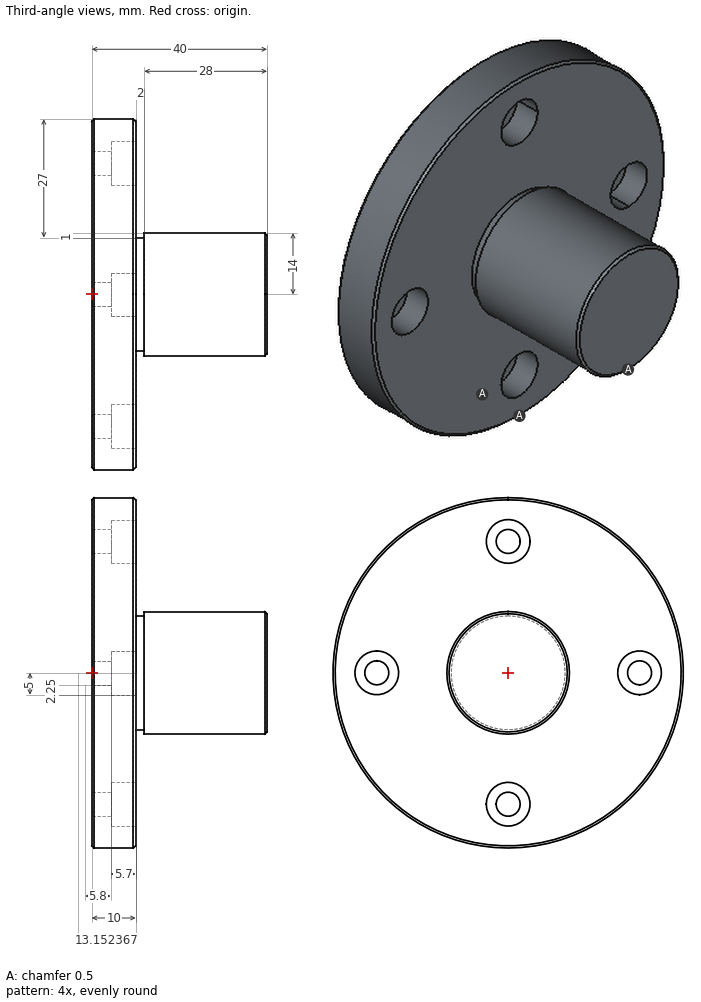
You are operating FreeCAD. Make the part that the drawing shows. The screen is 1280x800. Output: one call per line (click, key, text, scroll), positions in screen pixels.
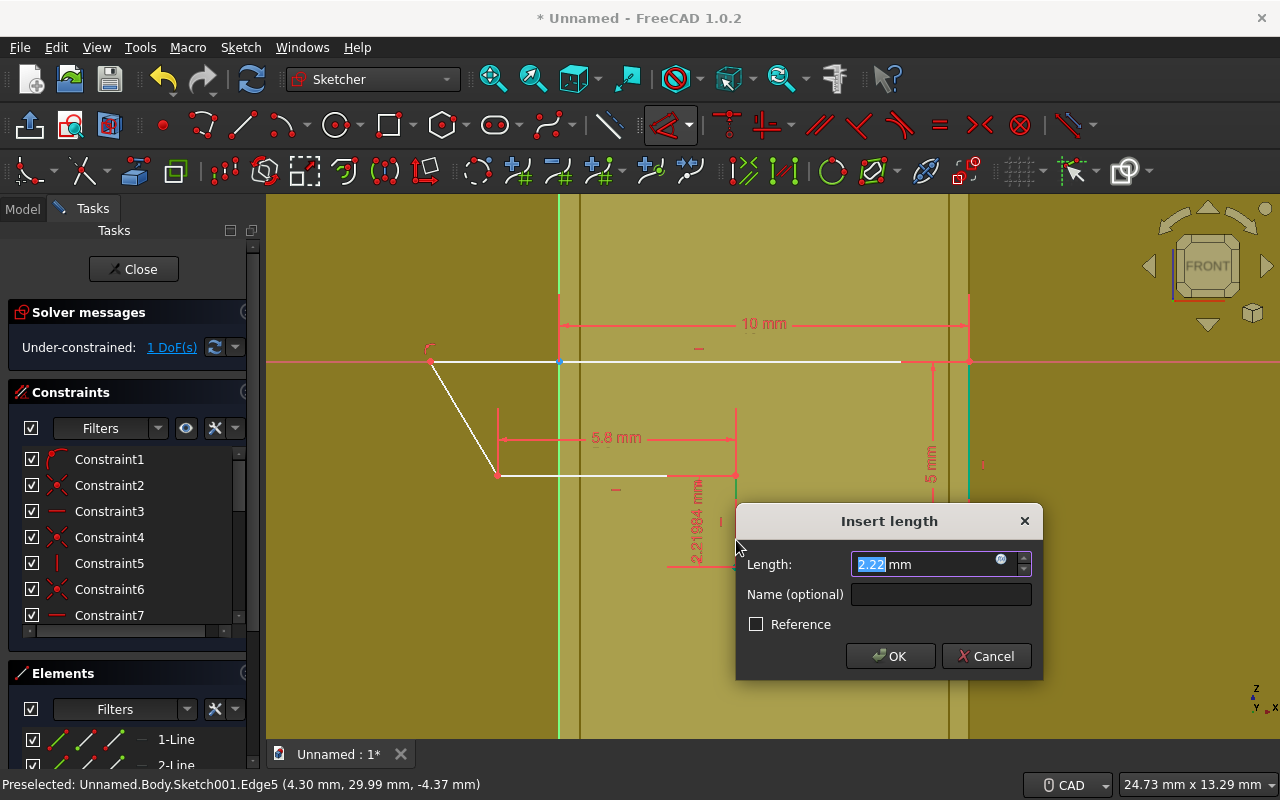
text(2.25)
key(Return)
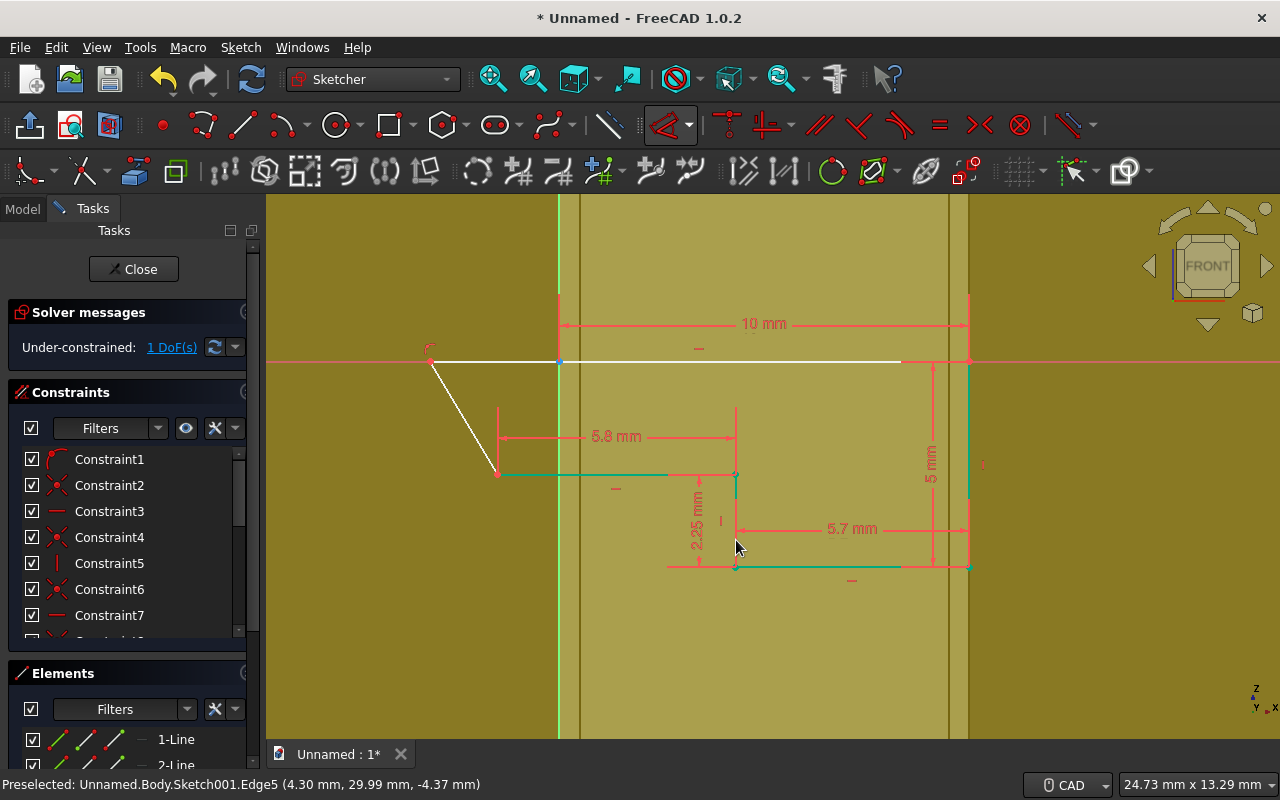
click(592, 362)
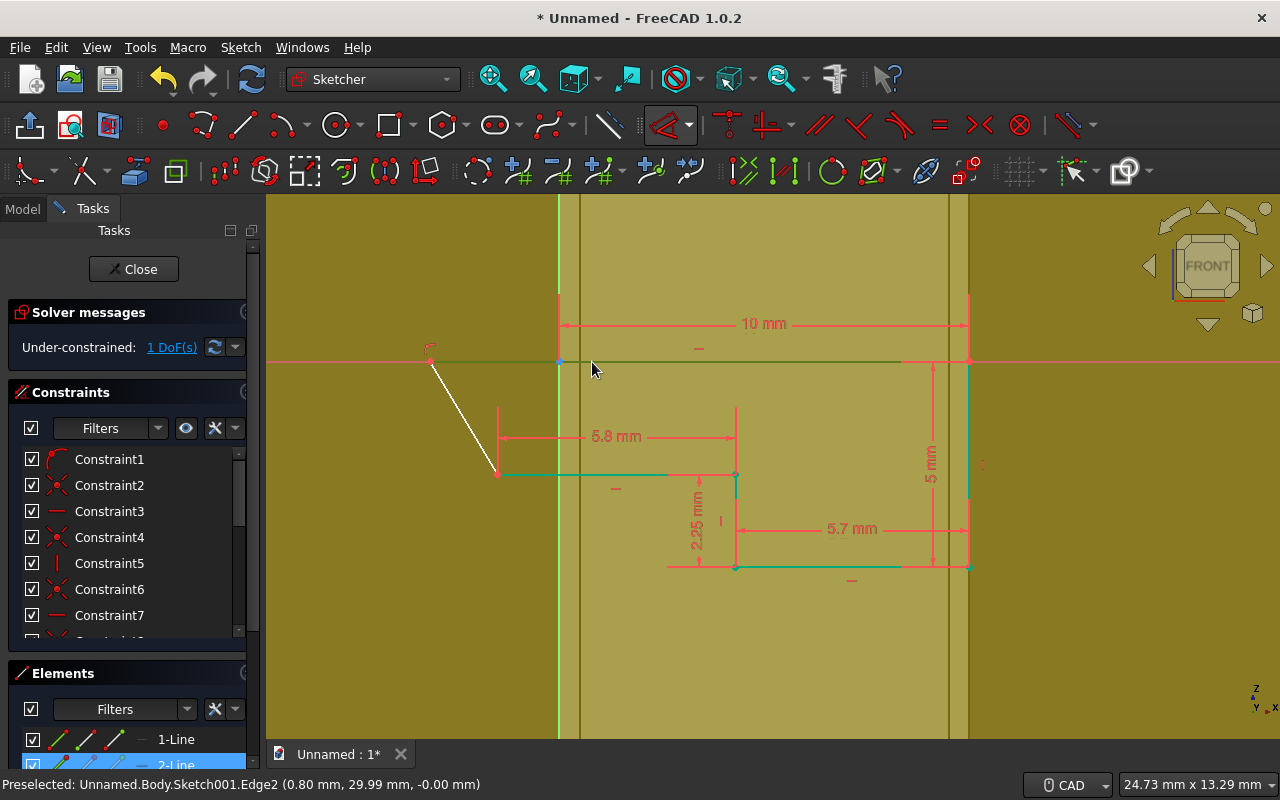
click(692, 126)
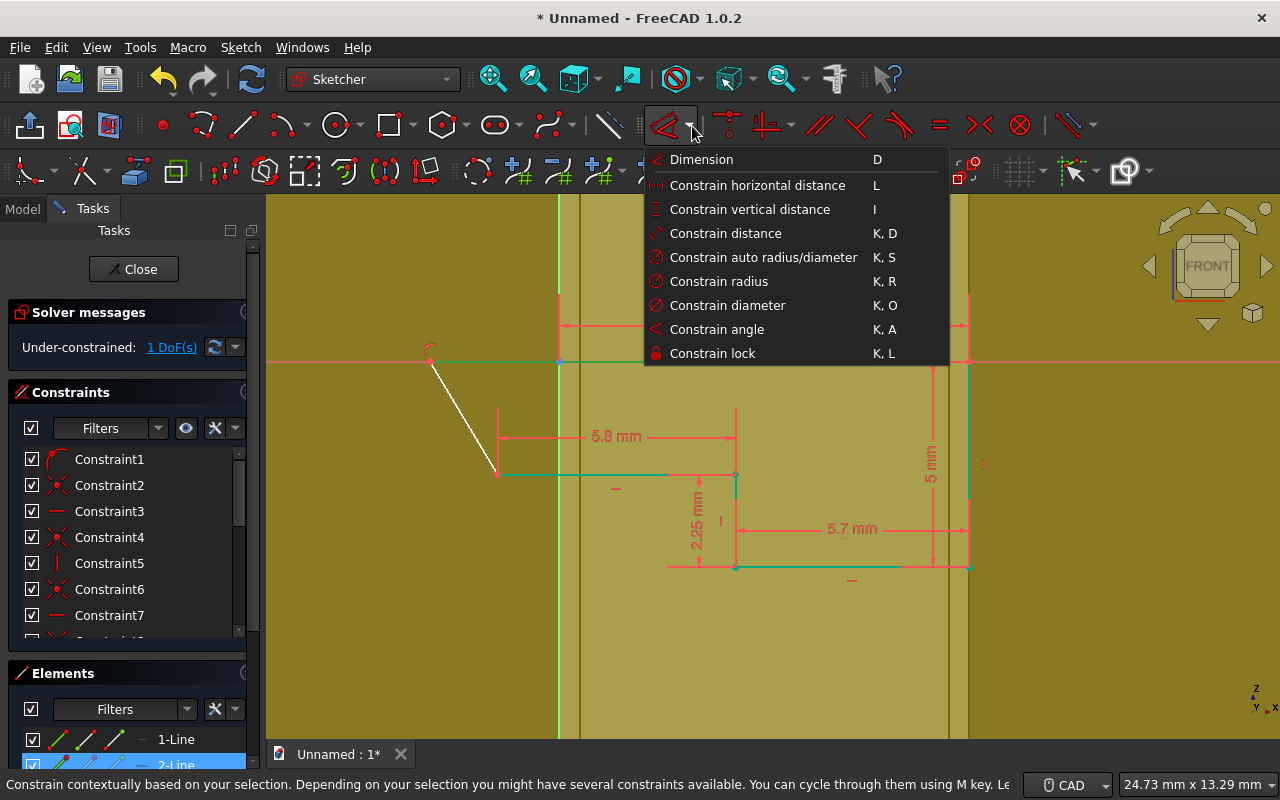
click(797, 185)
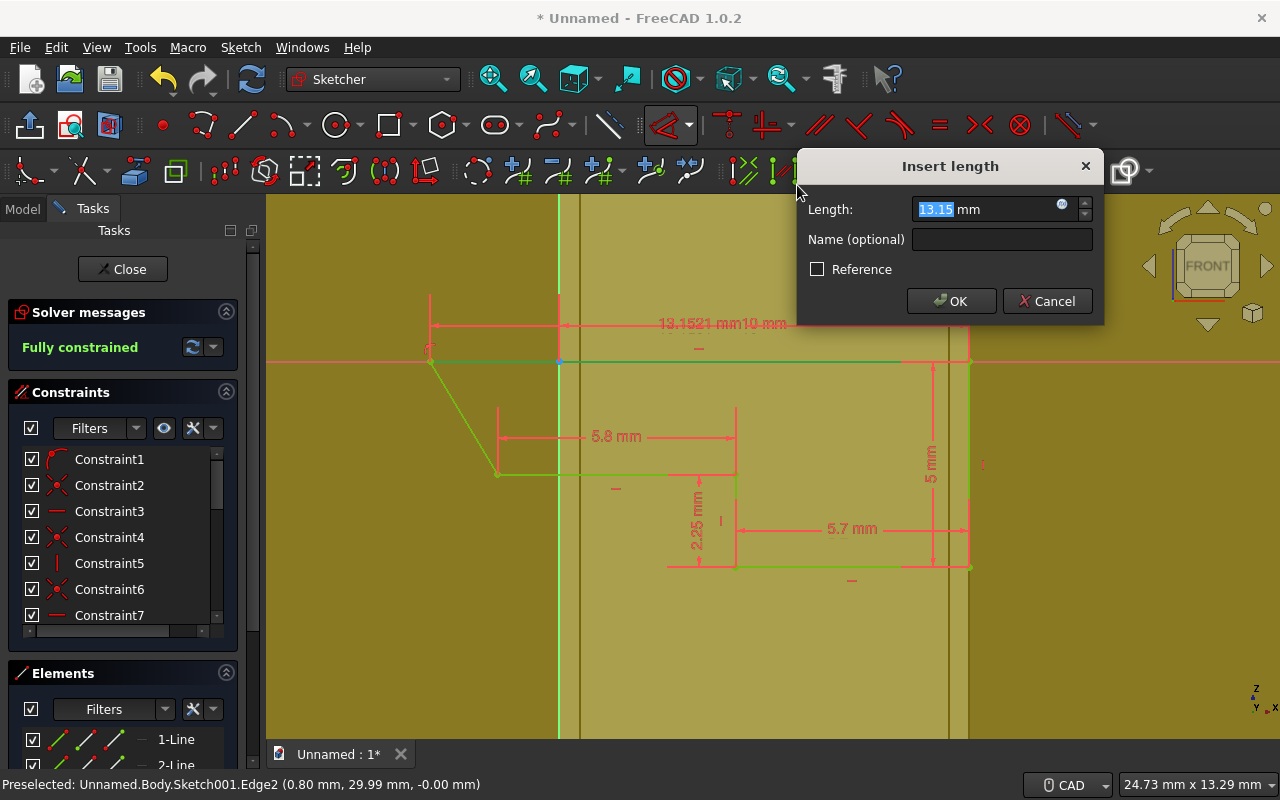
text(13.152367)
key(Return)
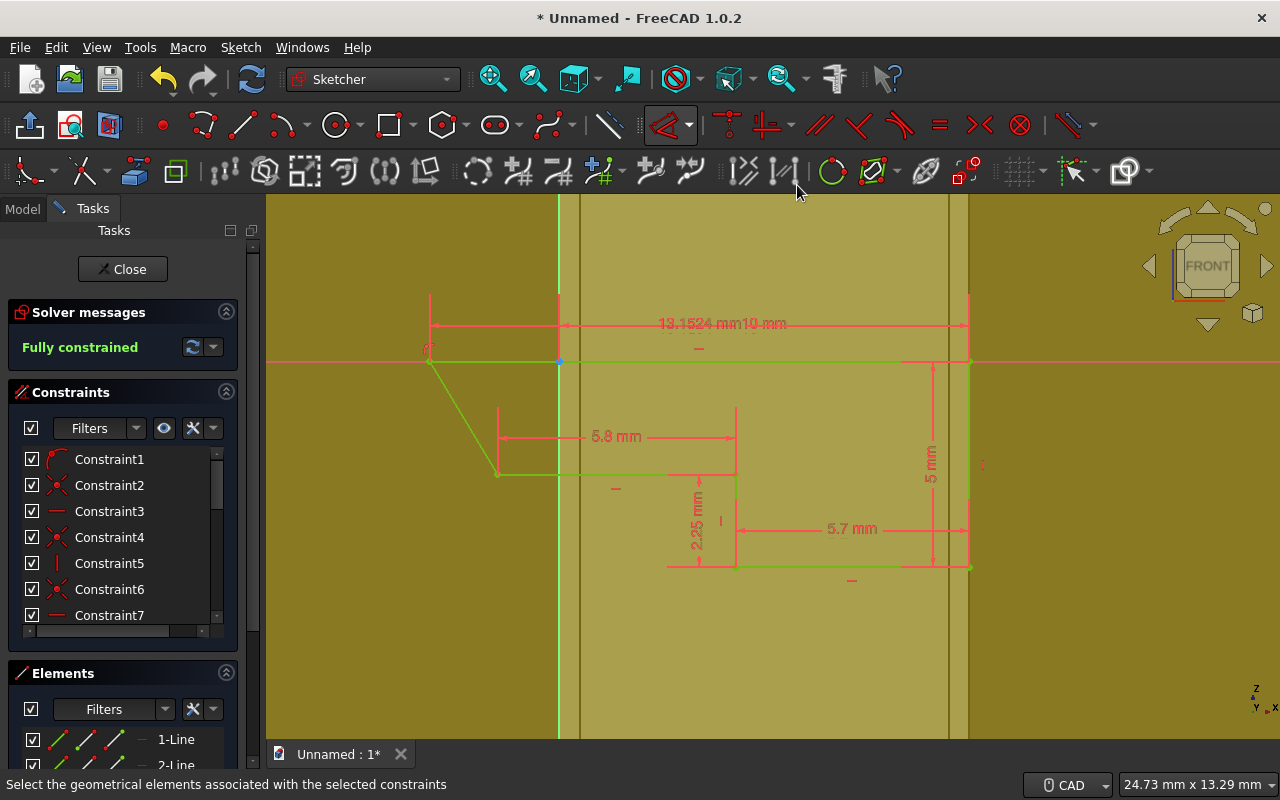
click(123, 269)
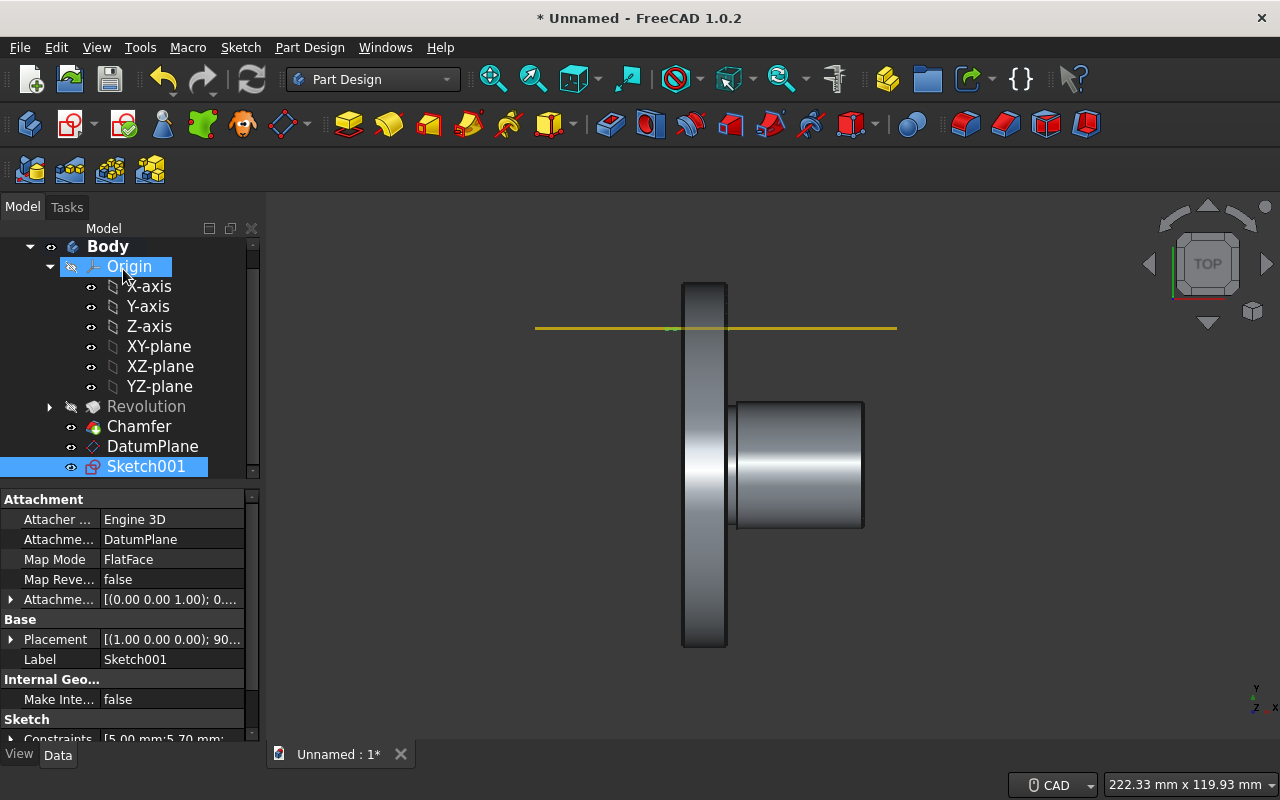
click(692, 124)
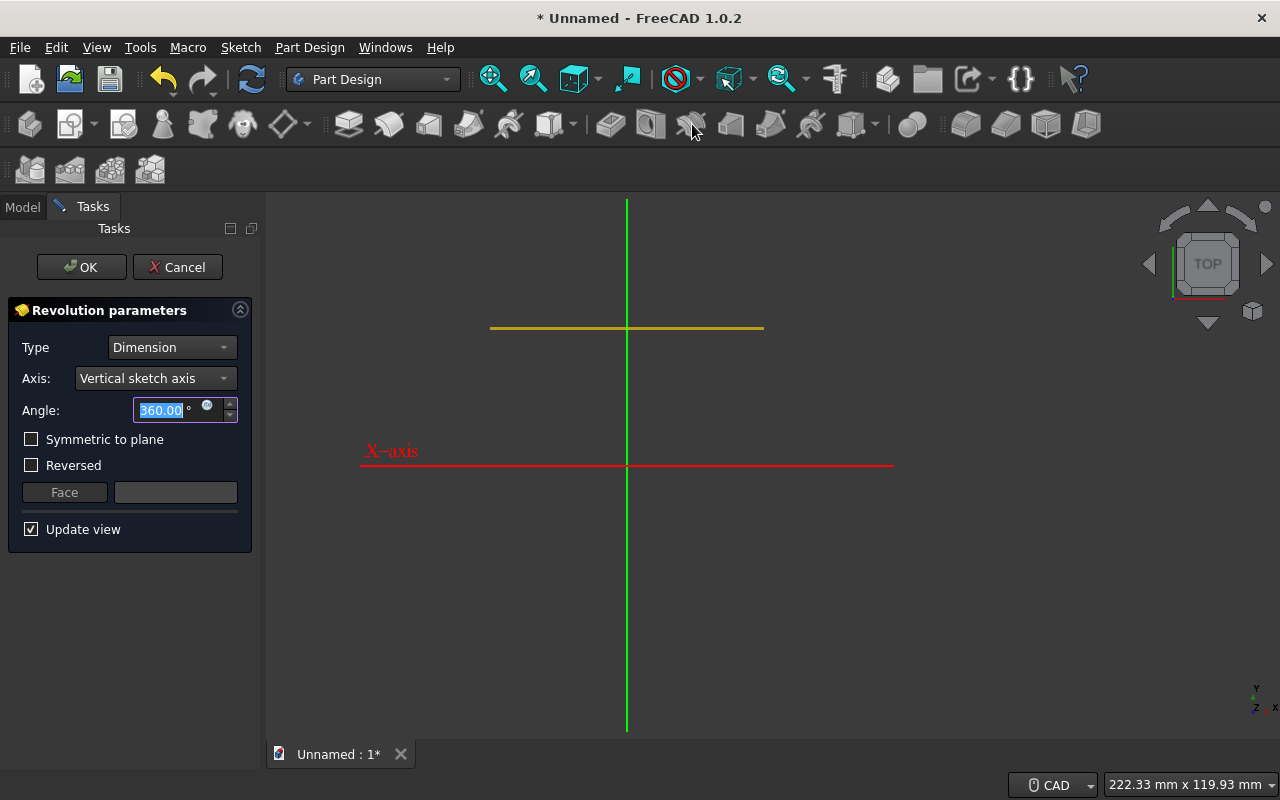
click(156, 378)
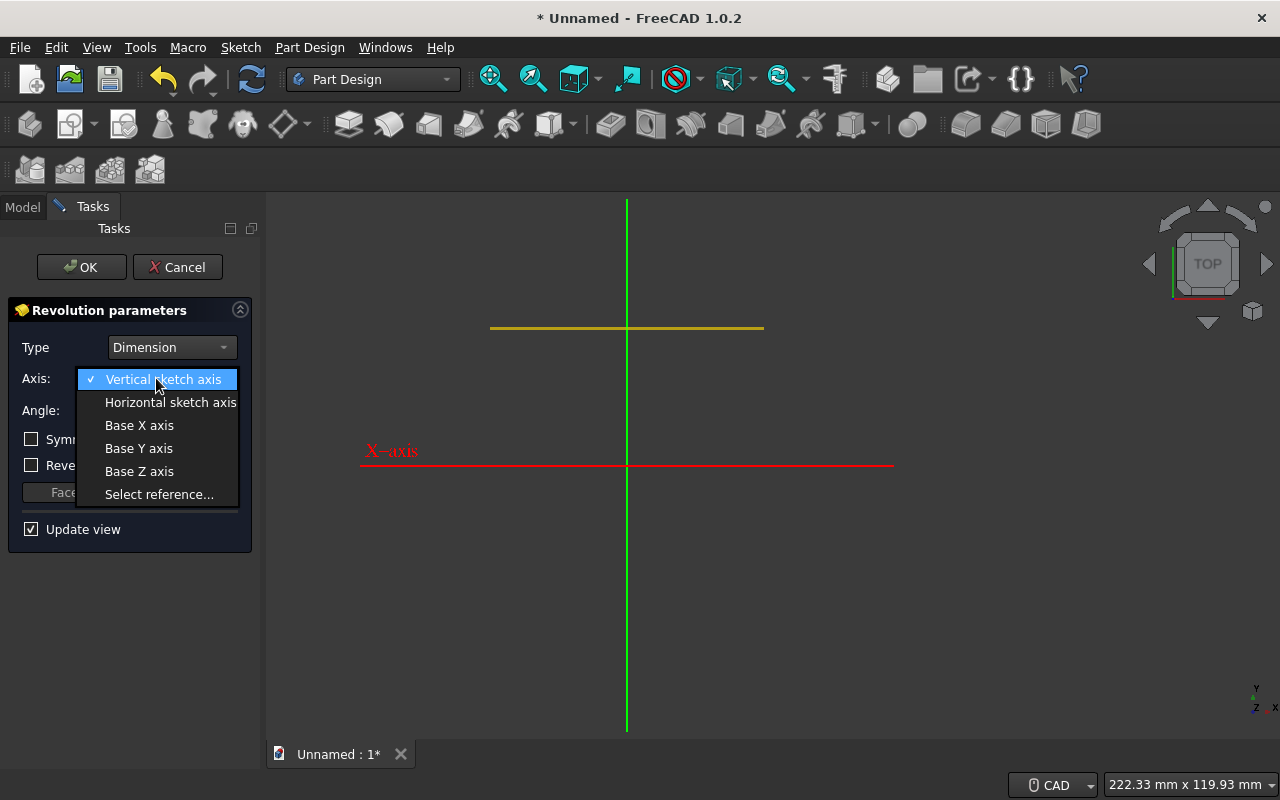
click(156, 402)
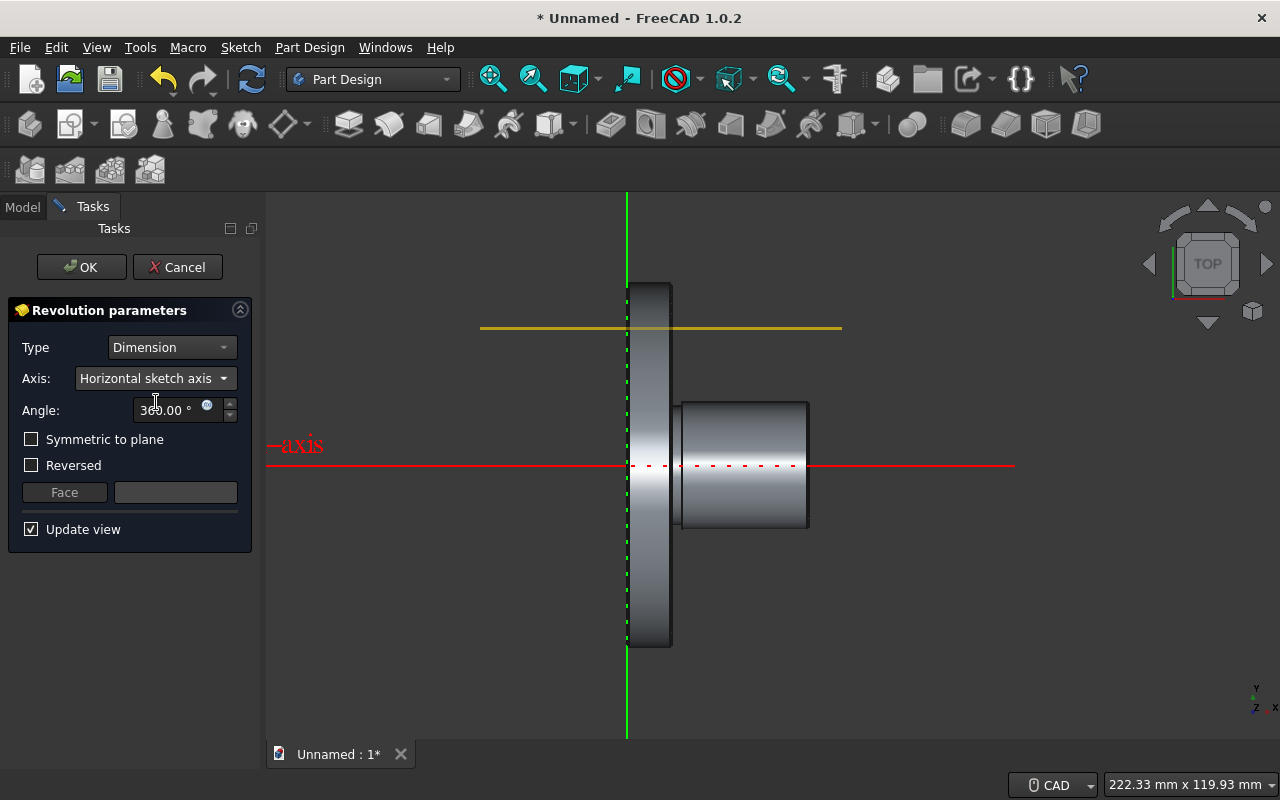
click(82, 267)